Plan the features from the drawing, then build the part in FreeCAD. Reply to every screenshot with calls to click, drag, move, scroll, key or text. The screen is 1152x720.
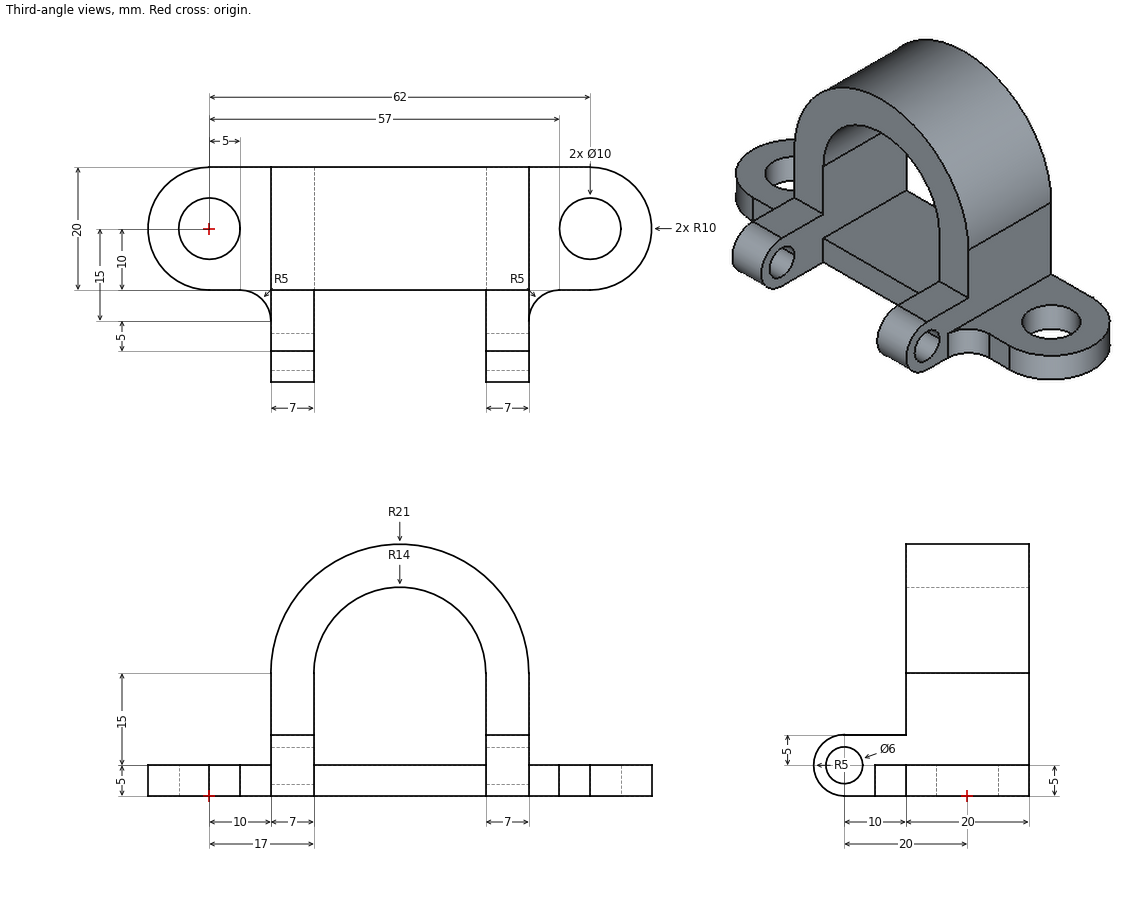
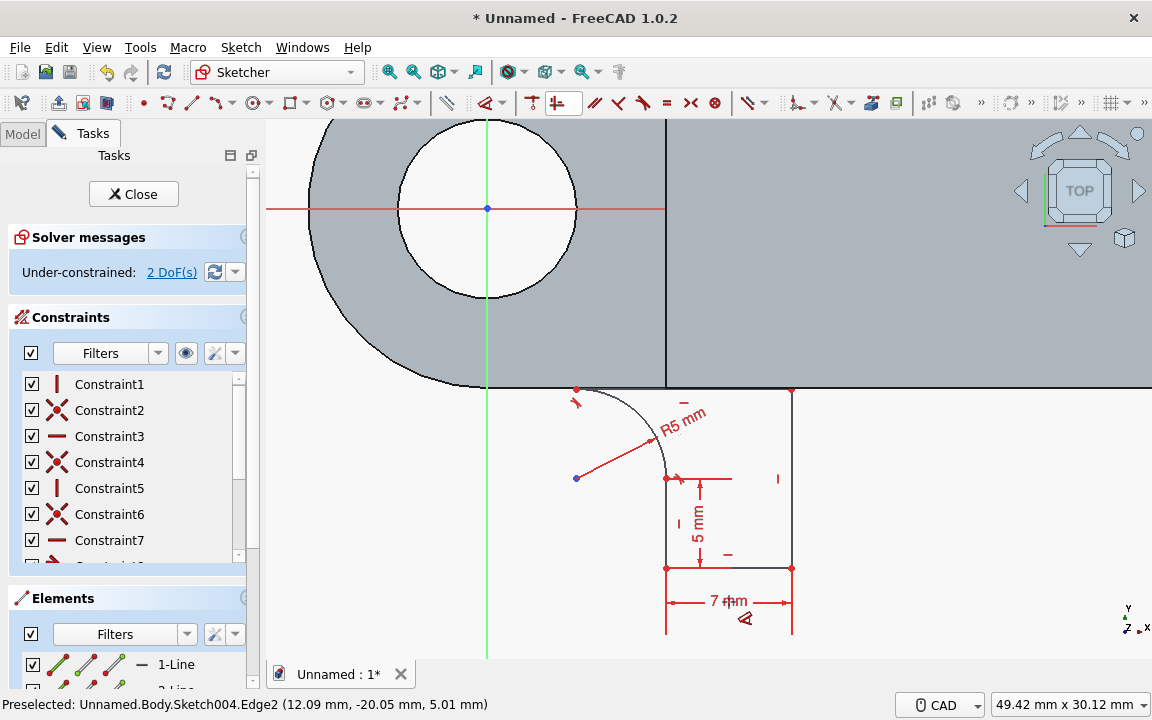
click(577, 389)
click(532, 175)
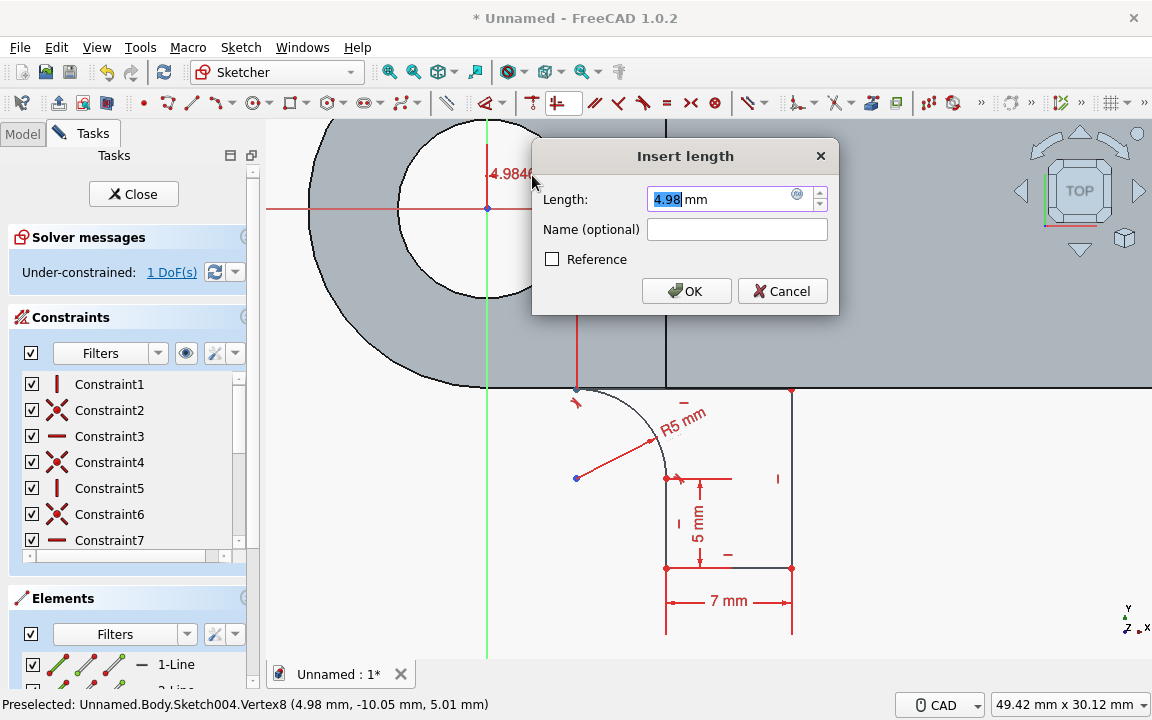
text(5)
key(Return)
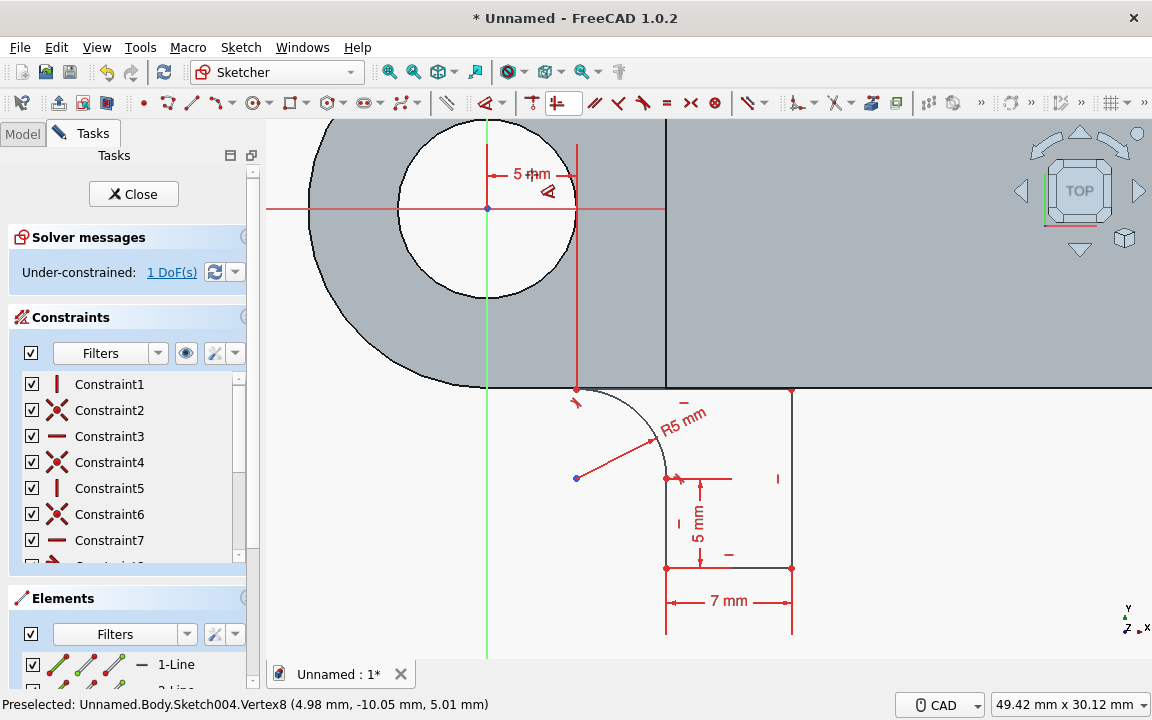
click(666, 479)
click(453, 344)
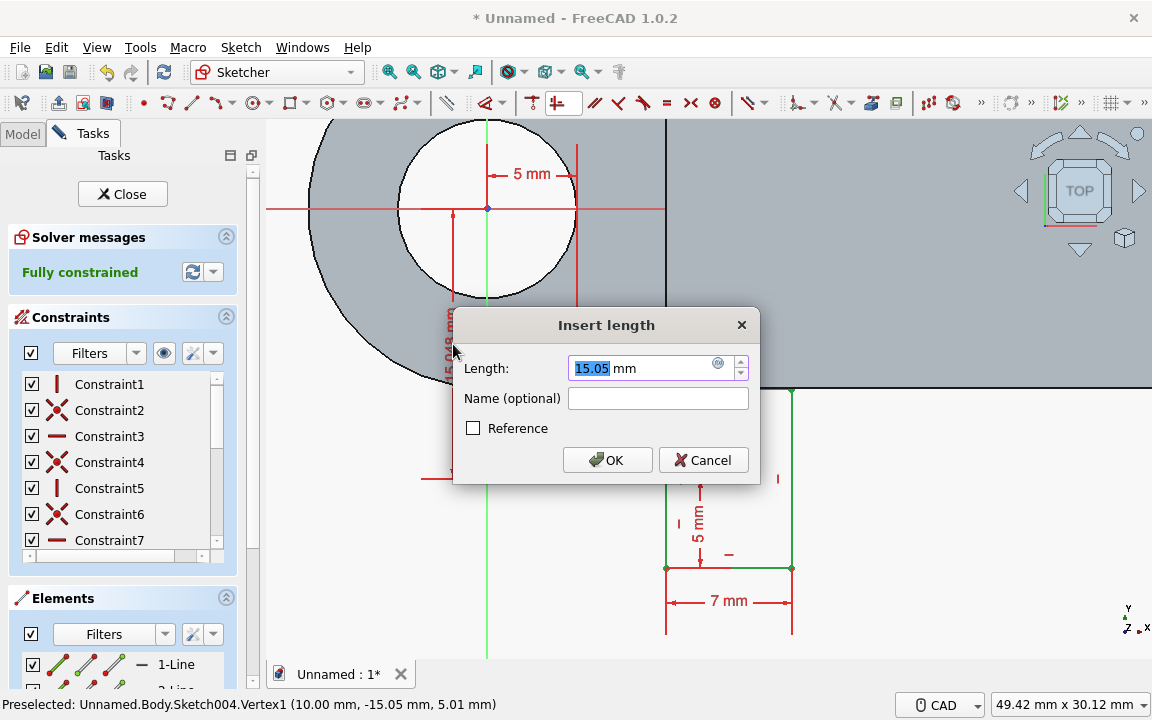
text(15)
key(Return)
key(Escape)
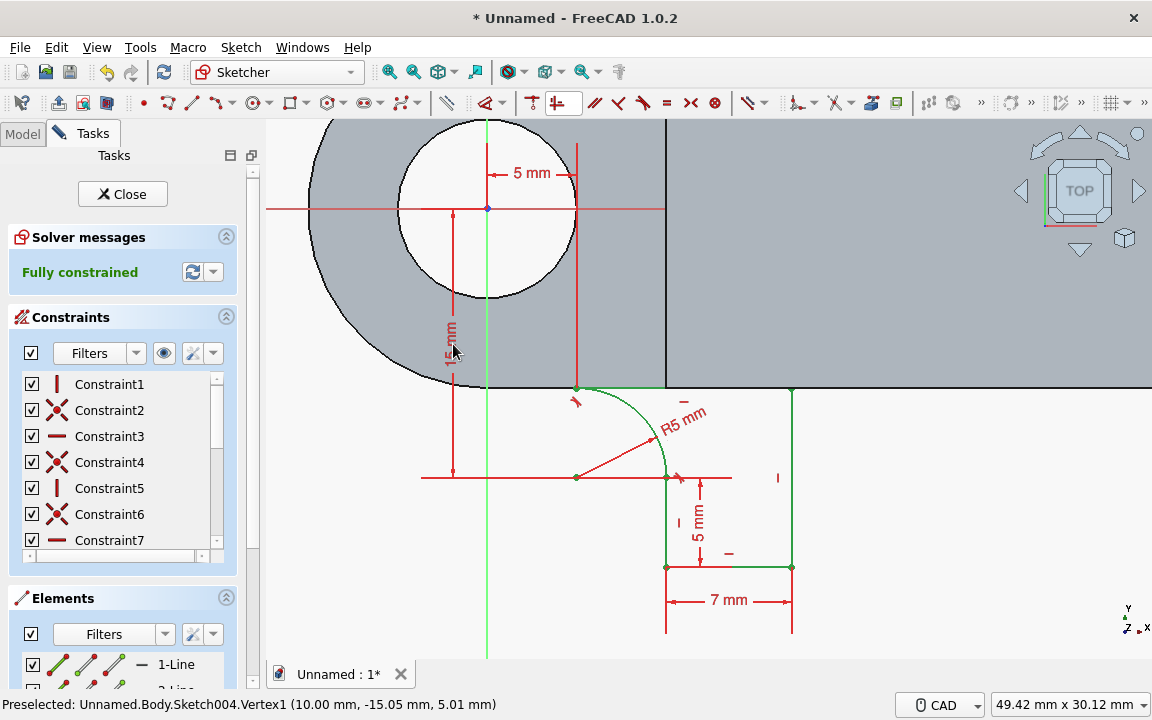
click(123, 194)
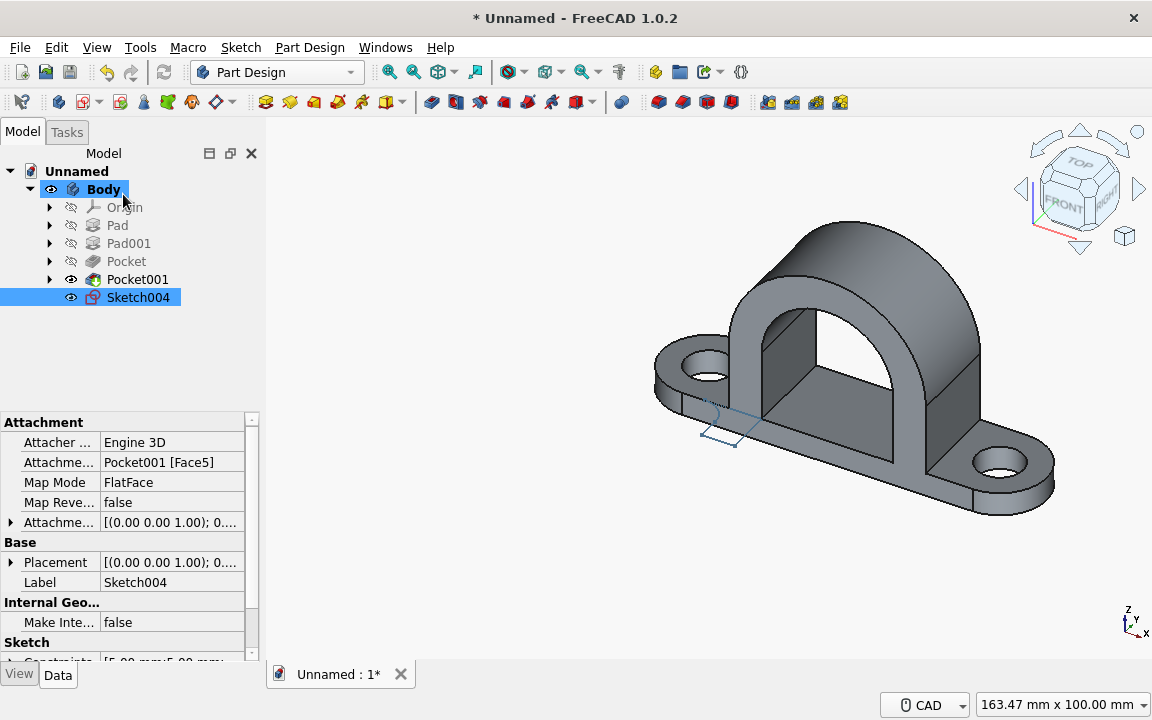
click(266, 102)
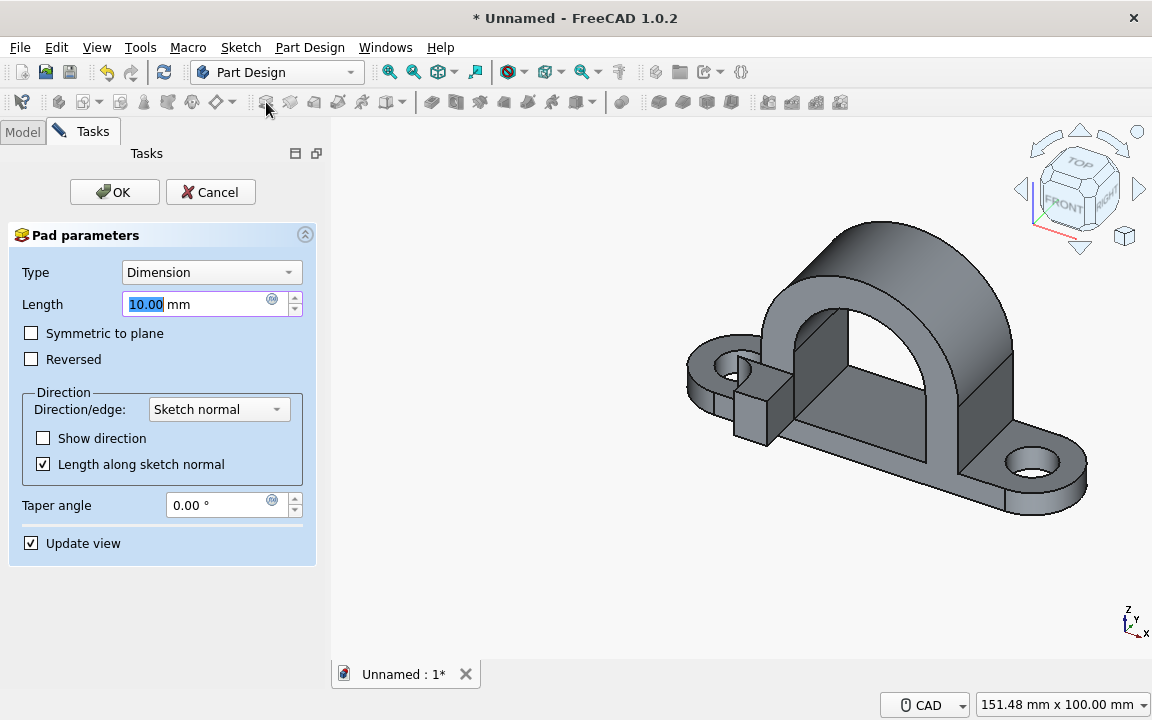
text(5)
key(Tab)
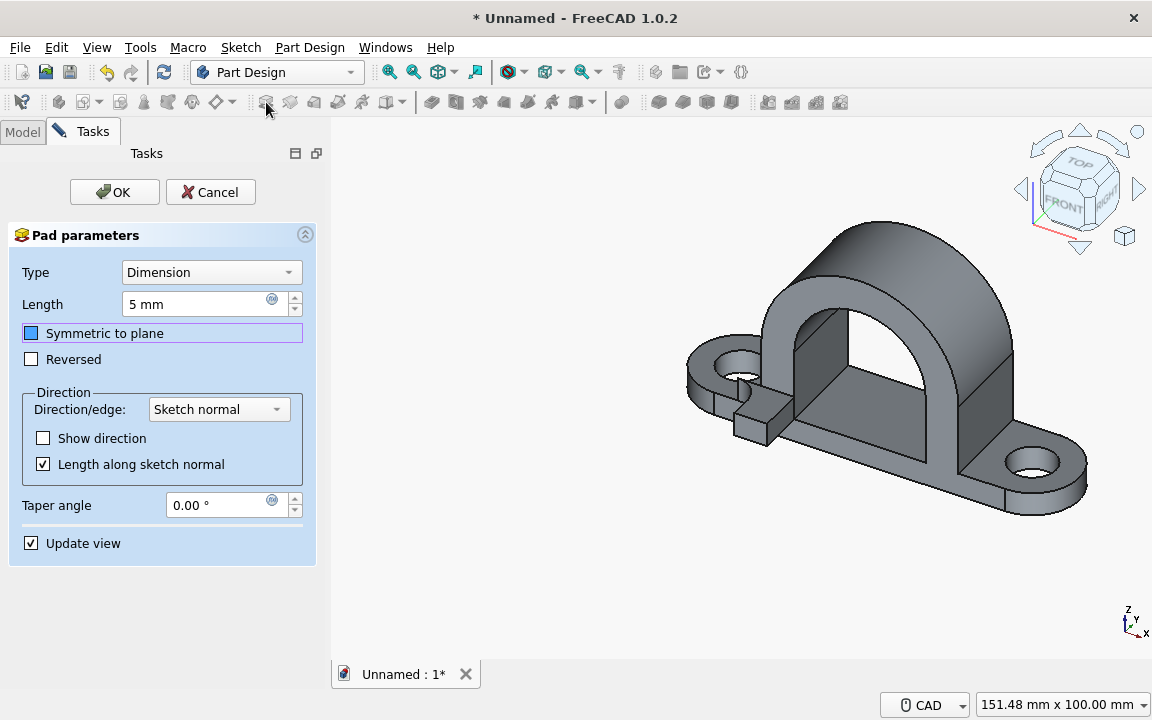
click(30, 359)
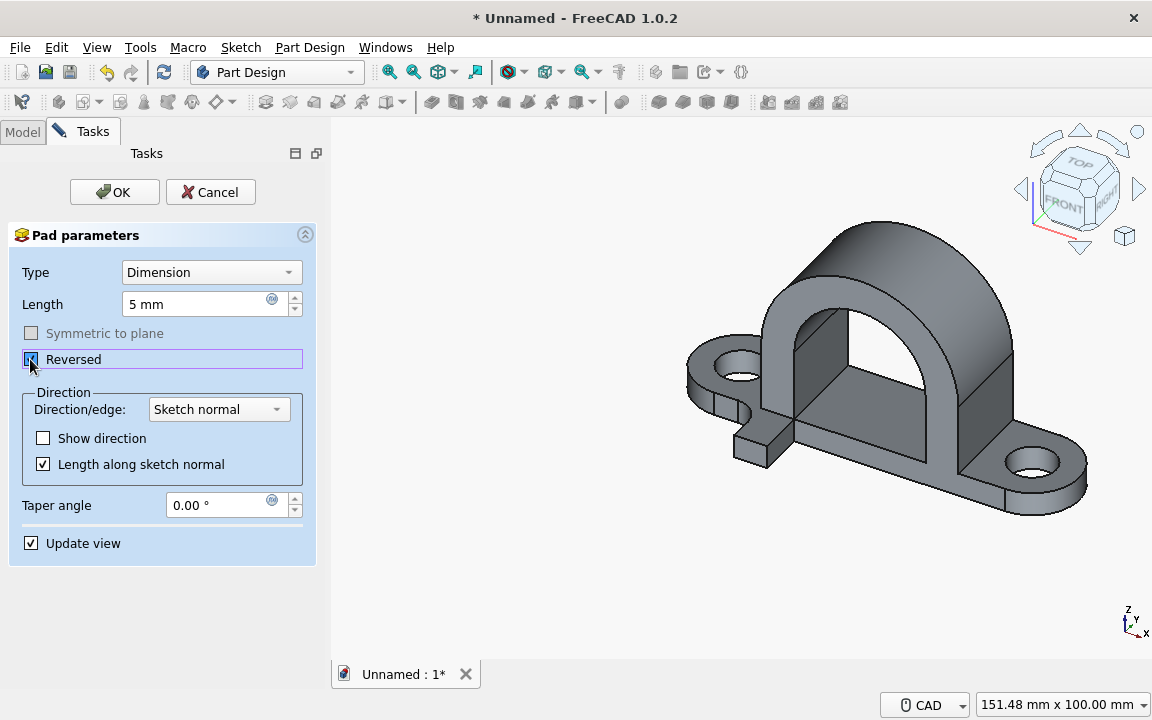
click(115, 192)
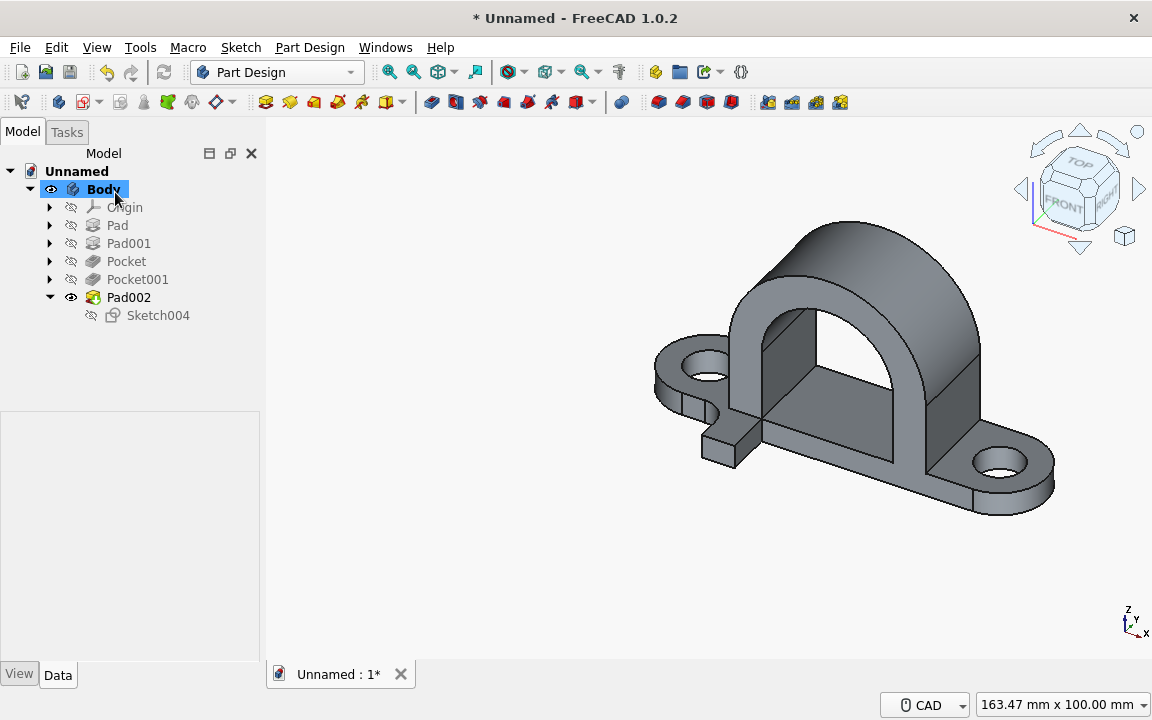
click(756, 438)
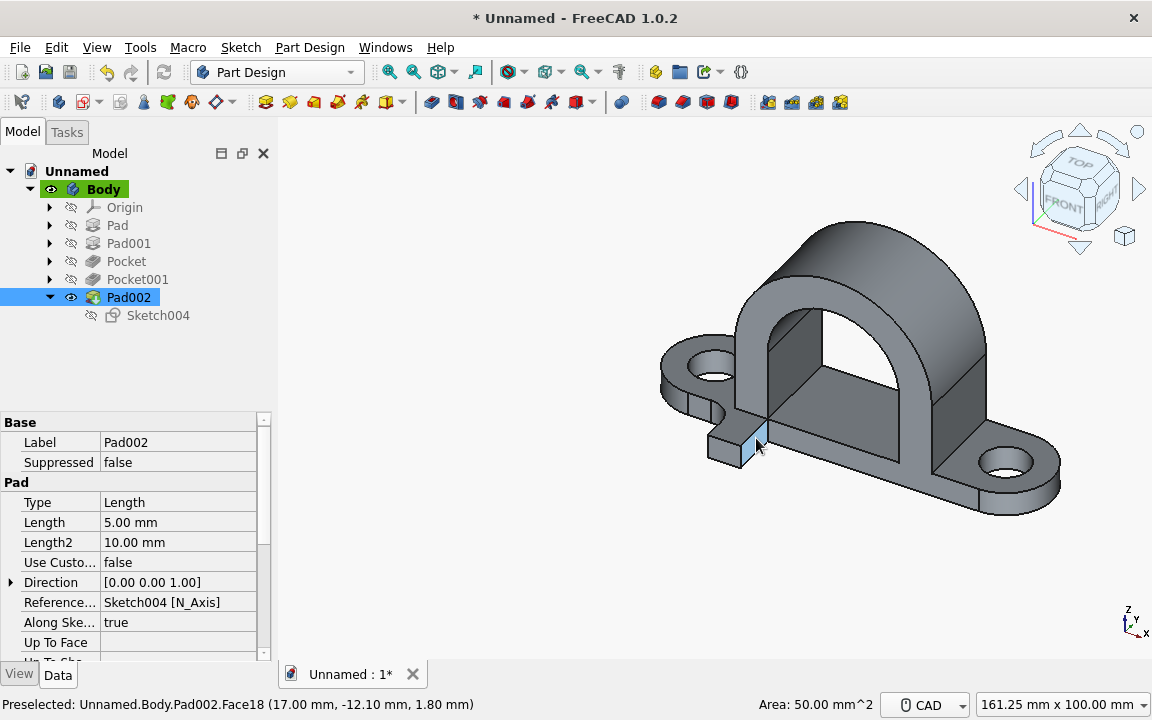
click(84, 102)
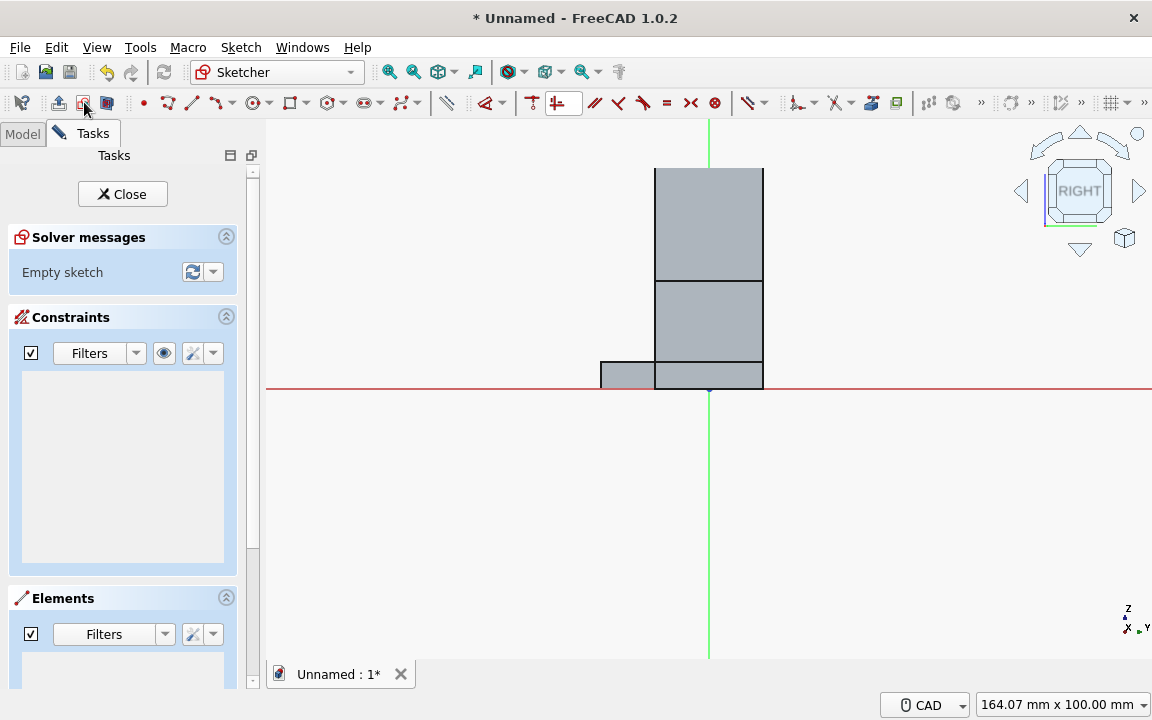
scroll(659, 355, up, 8)